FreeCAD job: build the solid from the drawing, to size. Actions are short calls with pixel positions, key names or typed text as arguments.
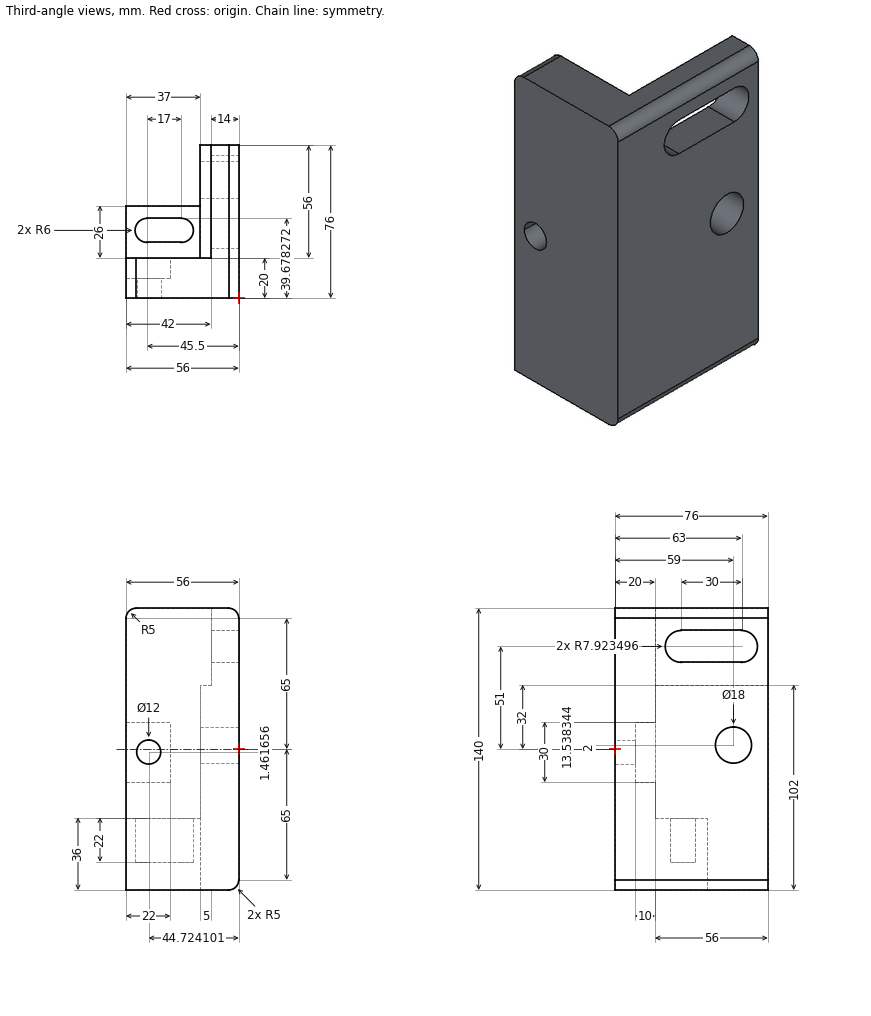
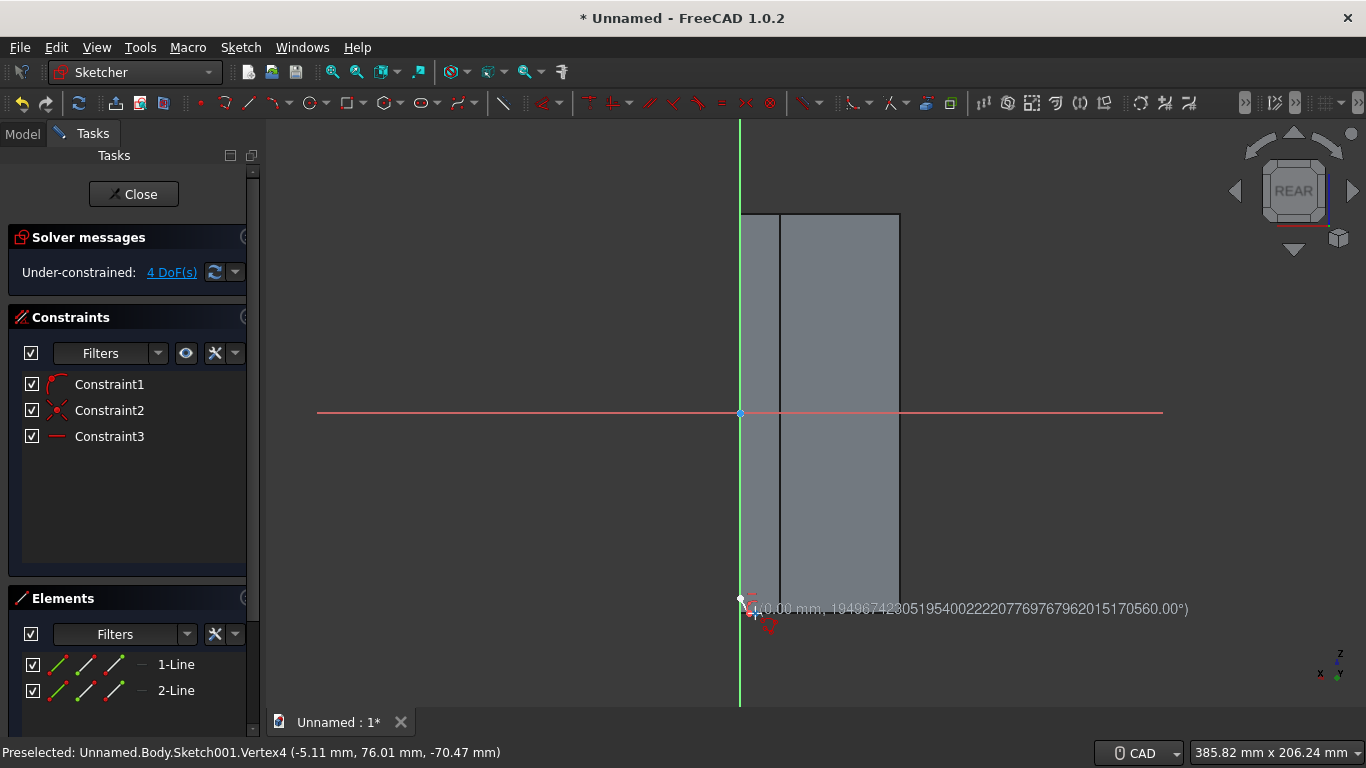
key(g)
key(3)
key(a)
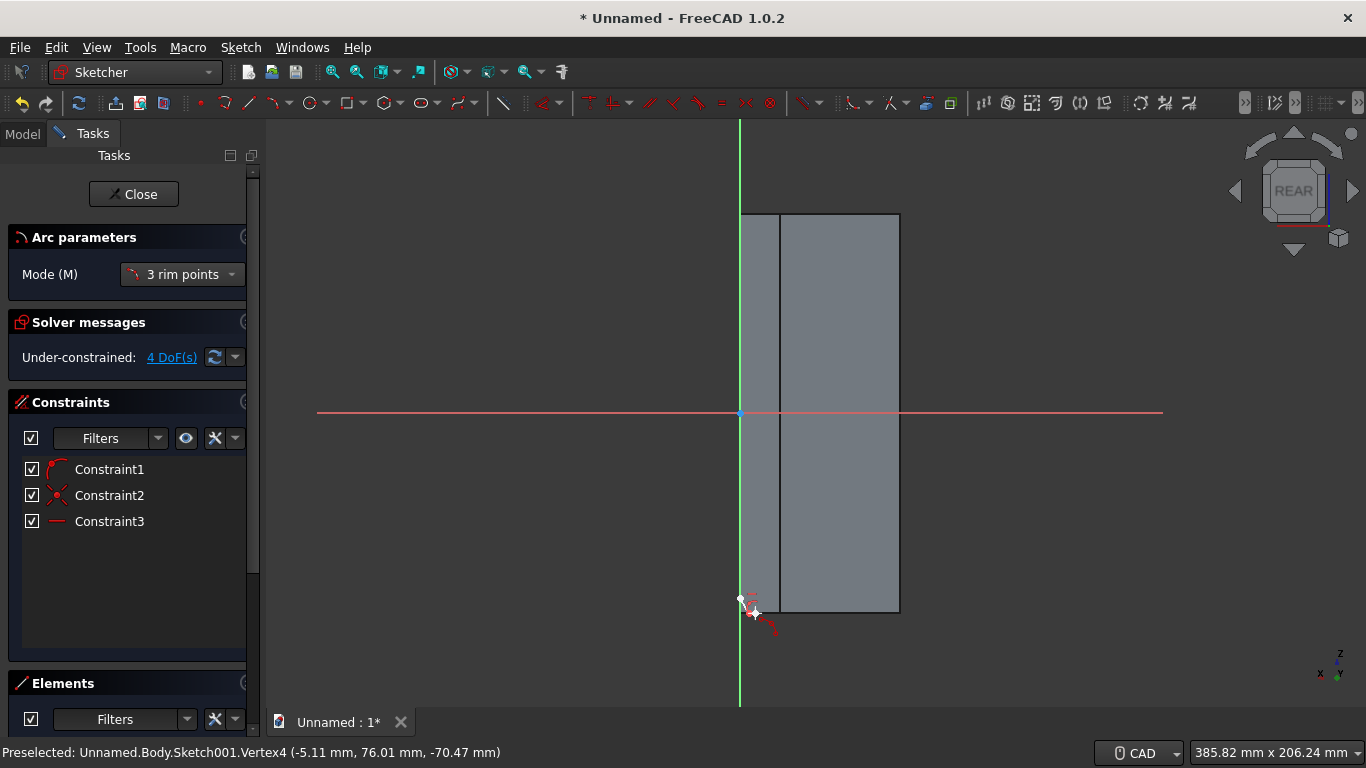
scroll(755, 613, up, 5)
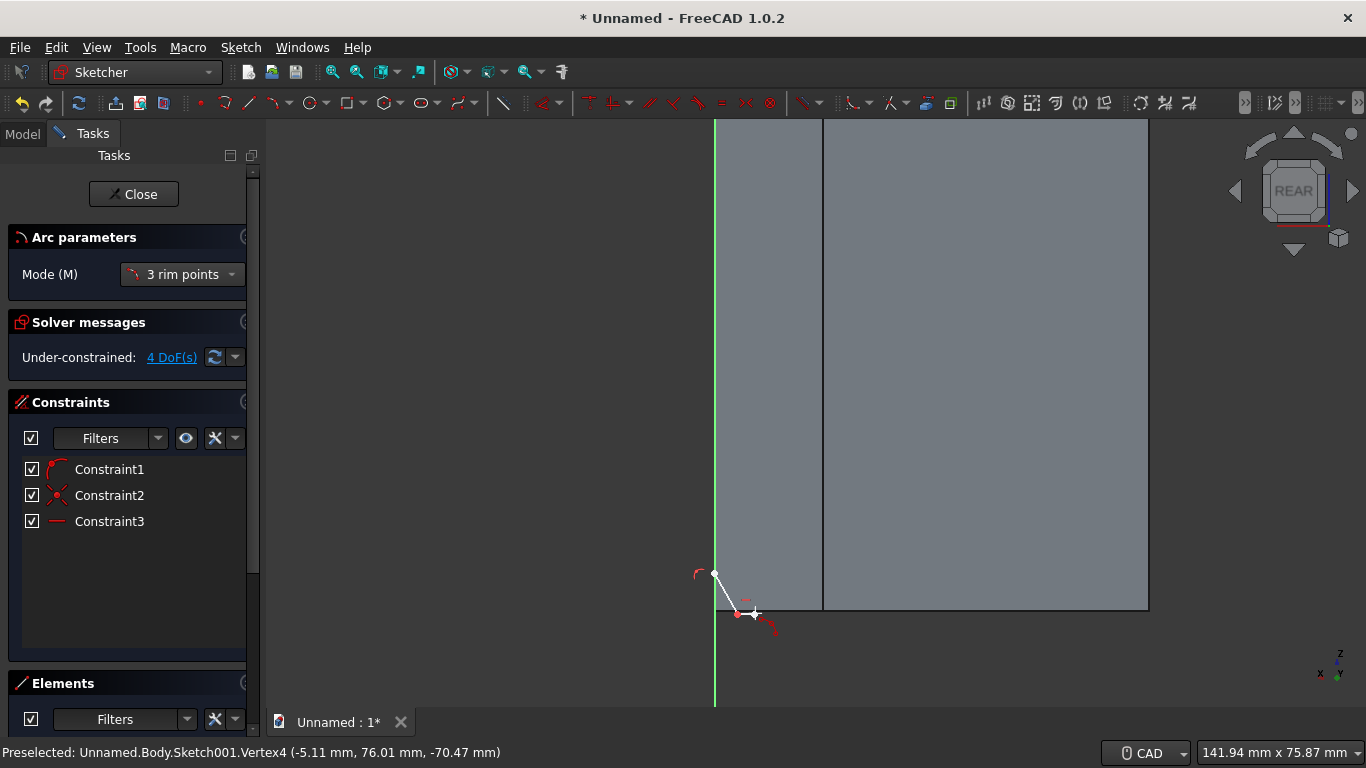
click(754, 614)
click(715, 573)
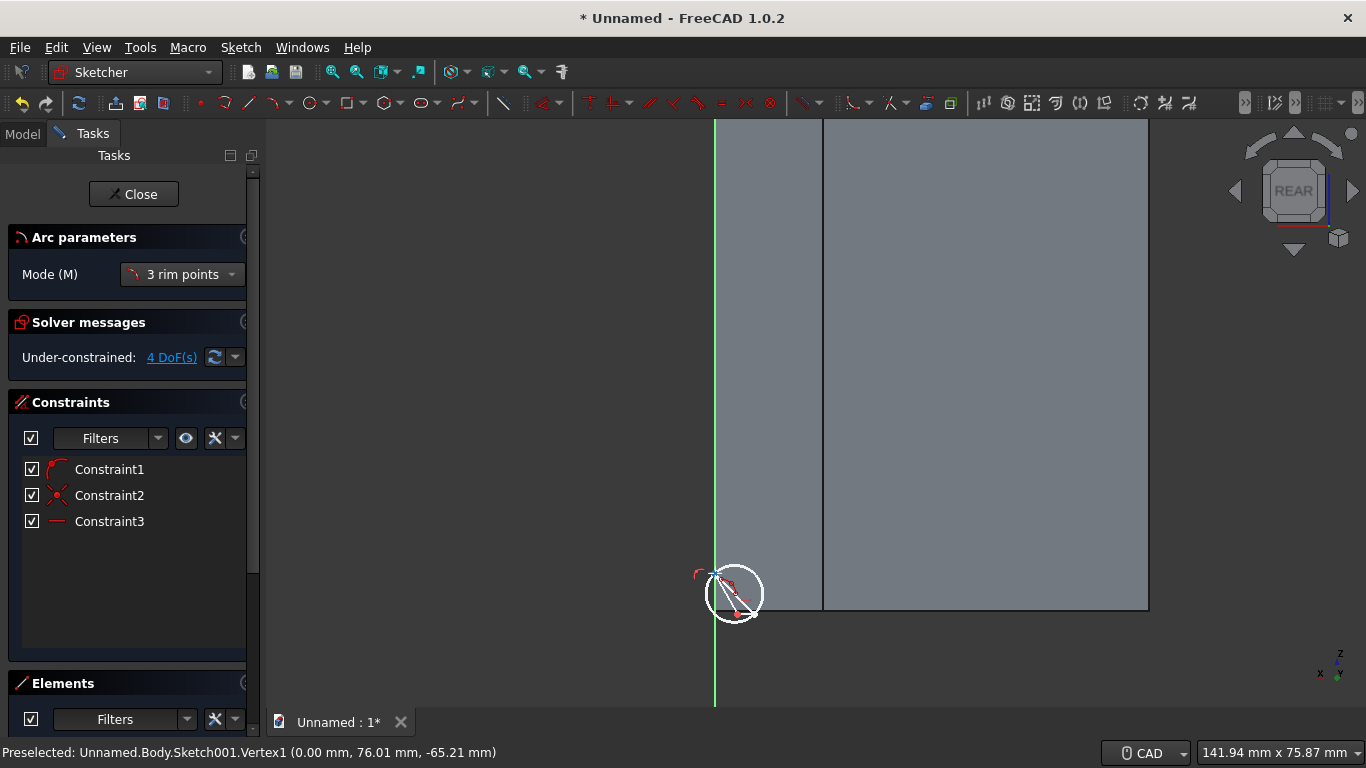
scroll(726, 599, up, 2)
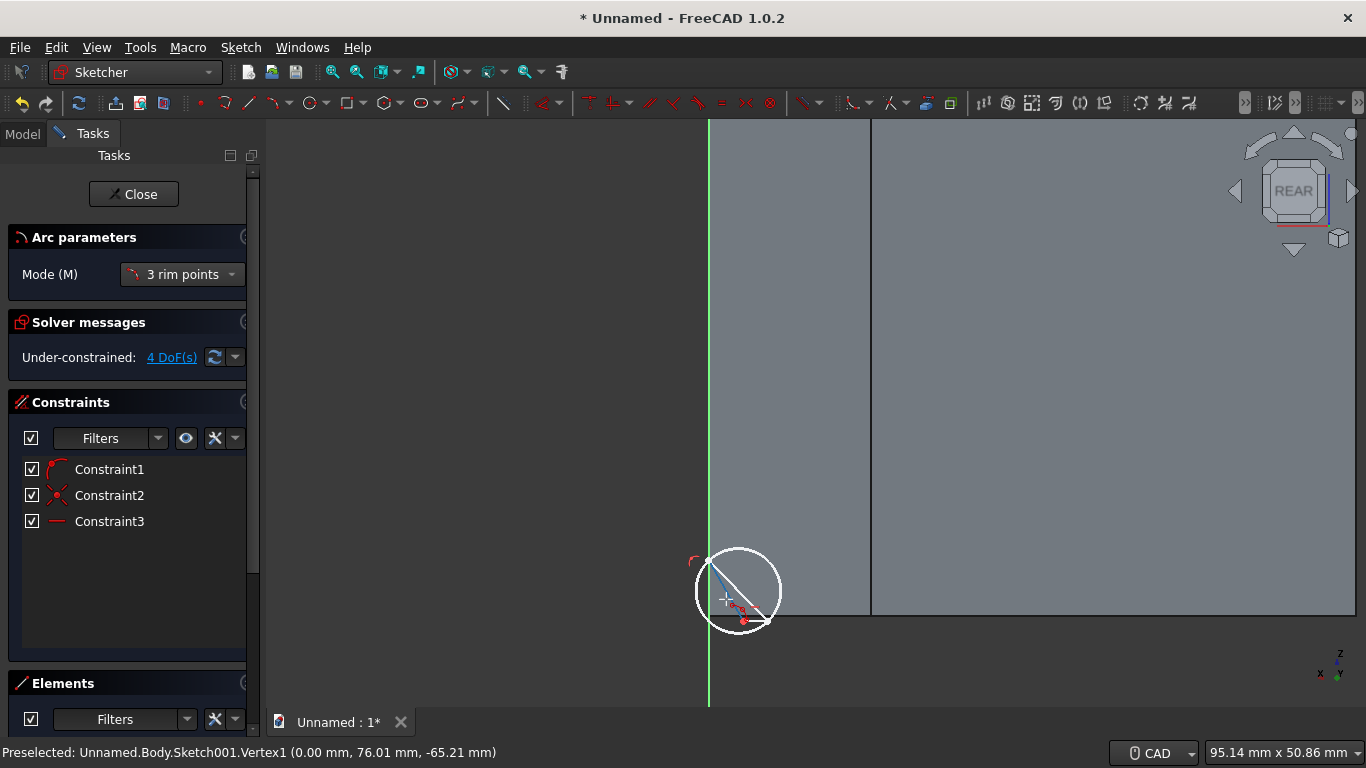
click(726, 599)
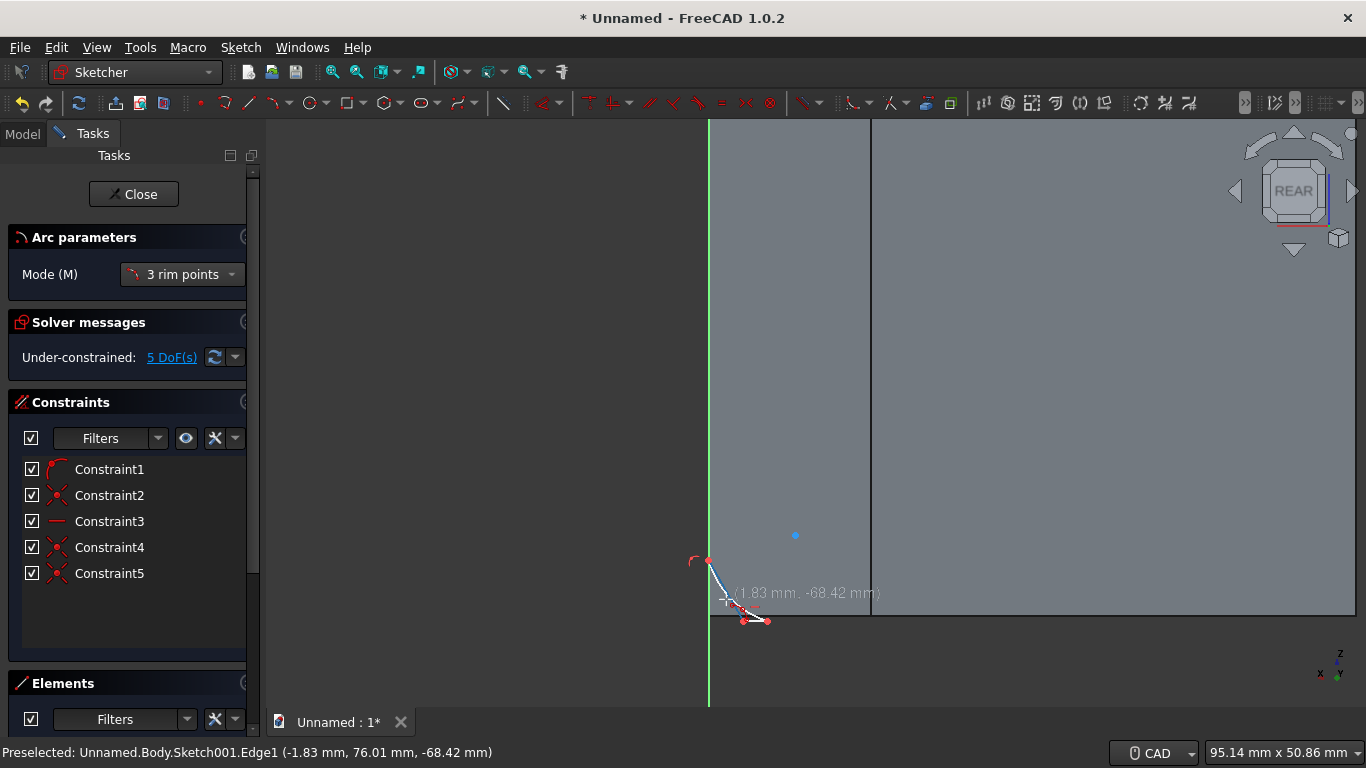
key(g)
key(m)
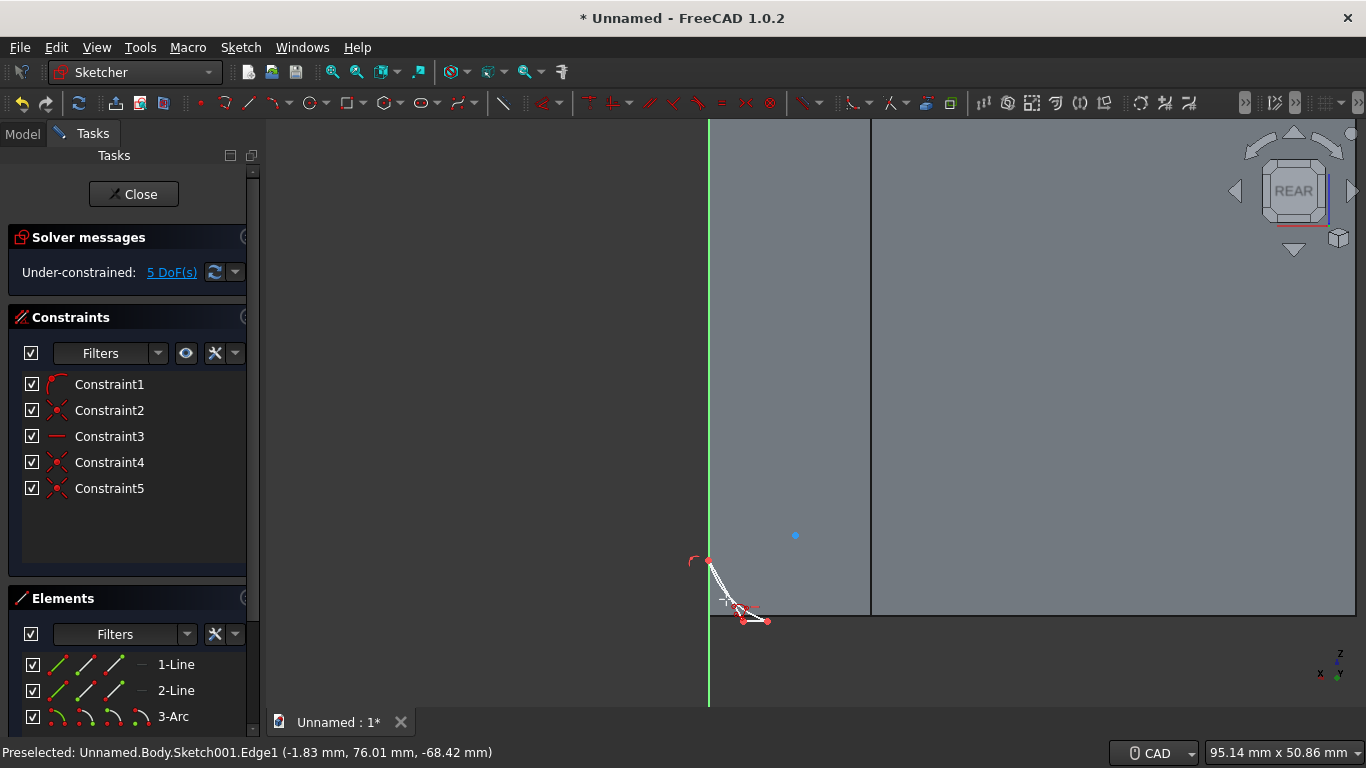
scroll(751, 611, down, 7)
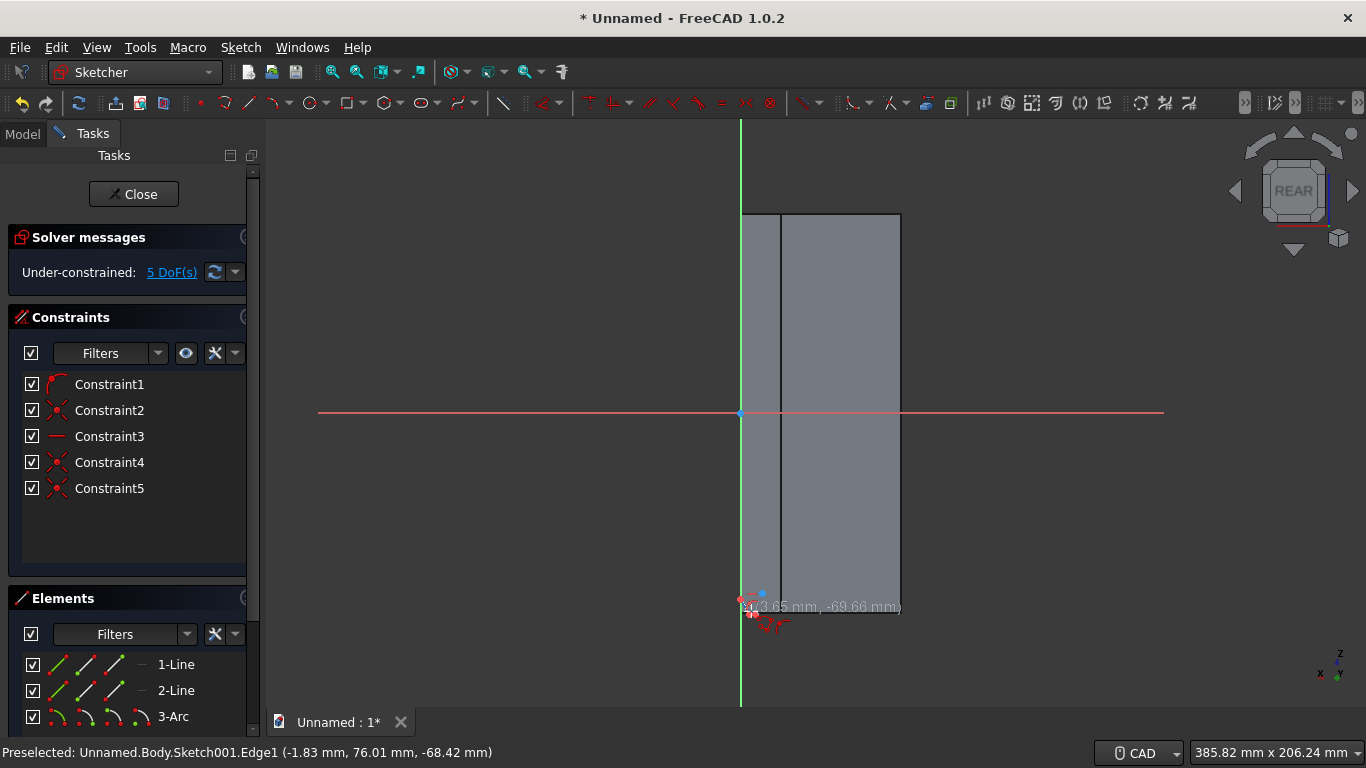
click(755, 214)
click(741, 214)
click(750, 228)
right_click(750, 228)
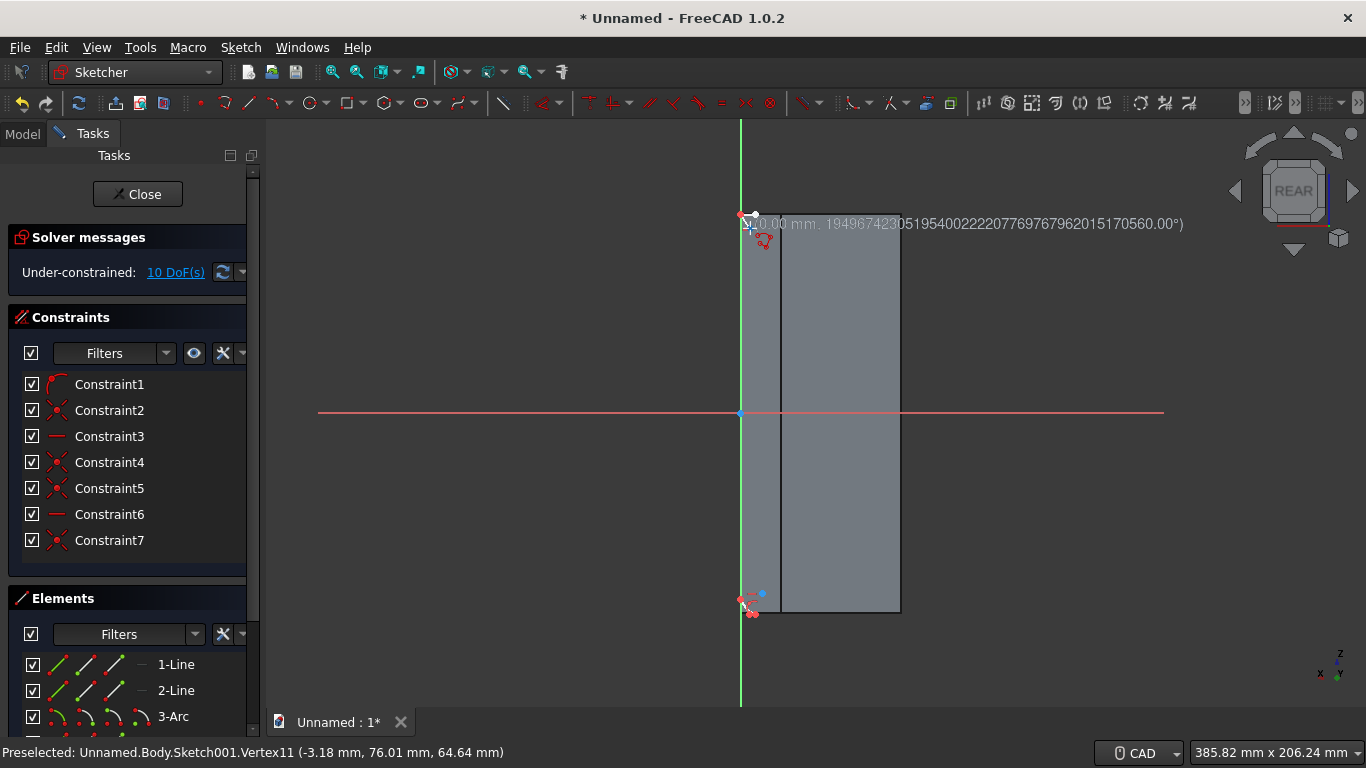
key(g)
key(3)
key(a)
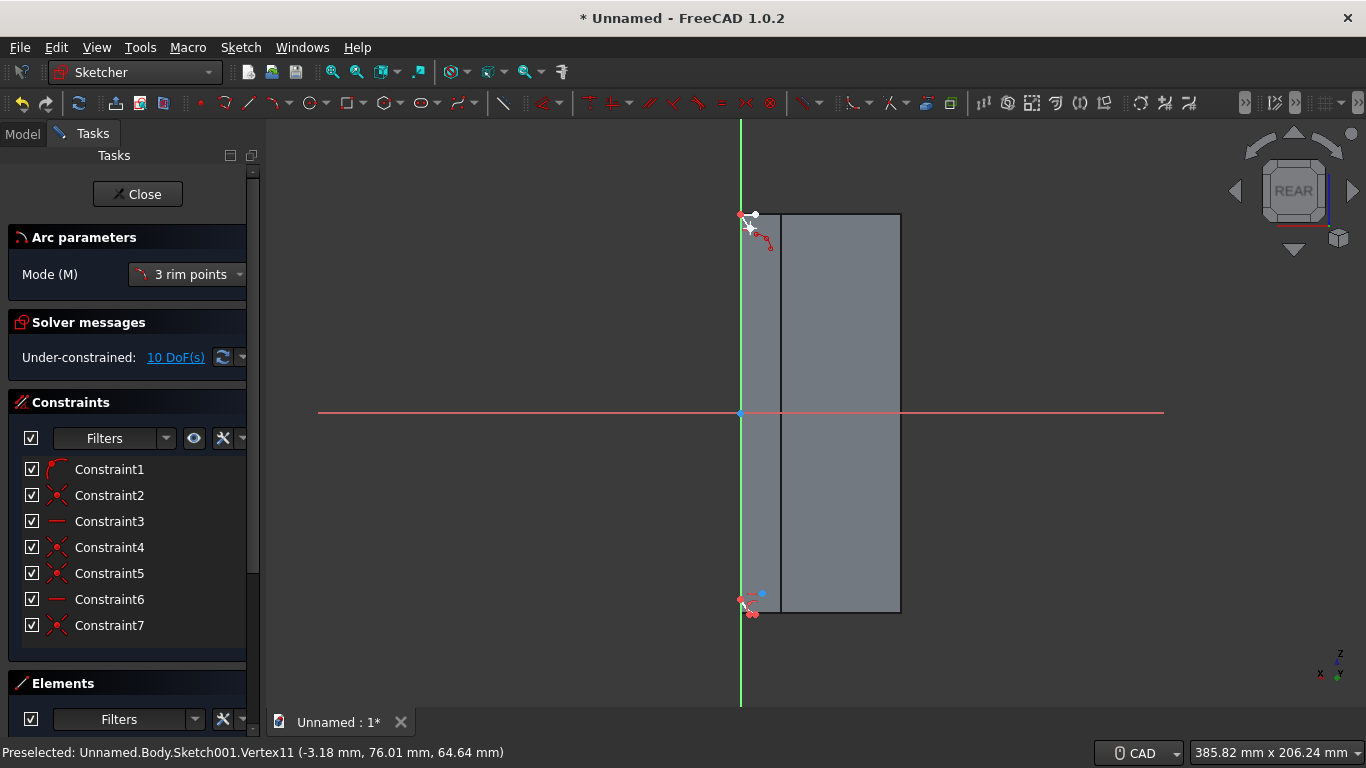
scroll(741, 228, up, 5)